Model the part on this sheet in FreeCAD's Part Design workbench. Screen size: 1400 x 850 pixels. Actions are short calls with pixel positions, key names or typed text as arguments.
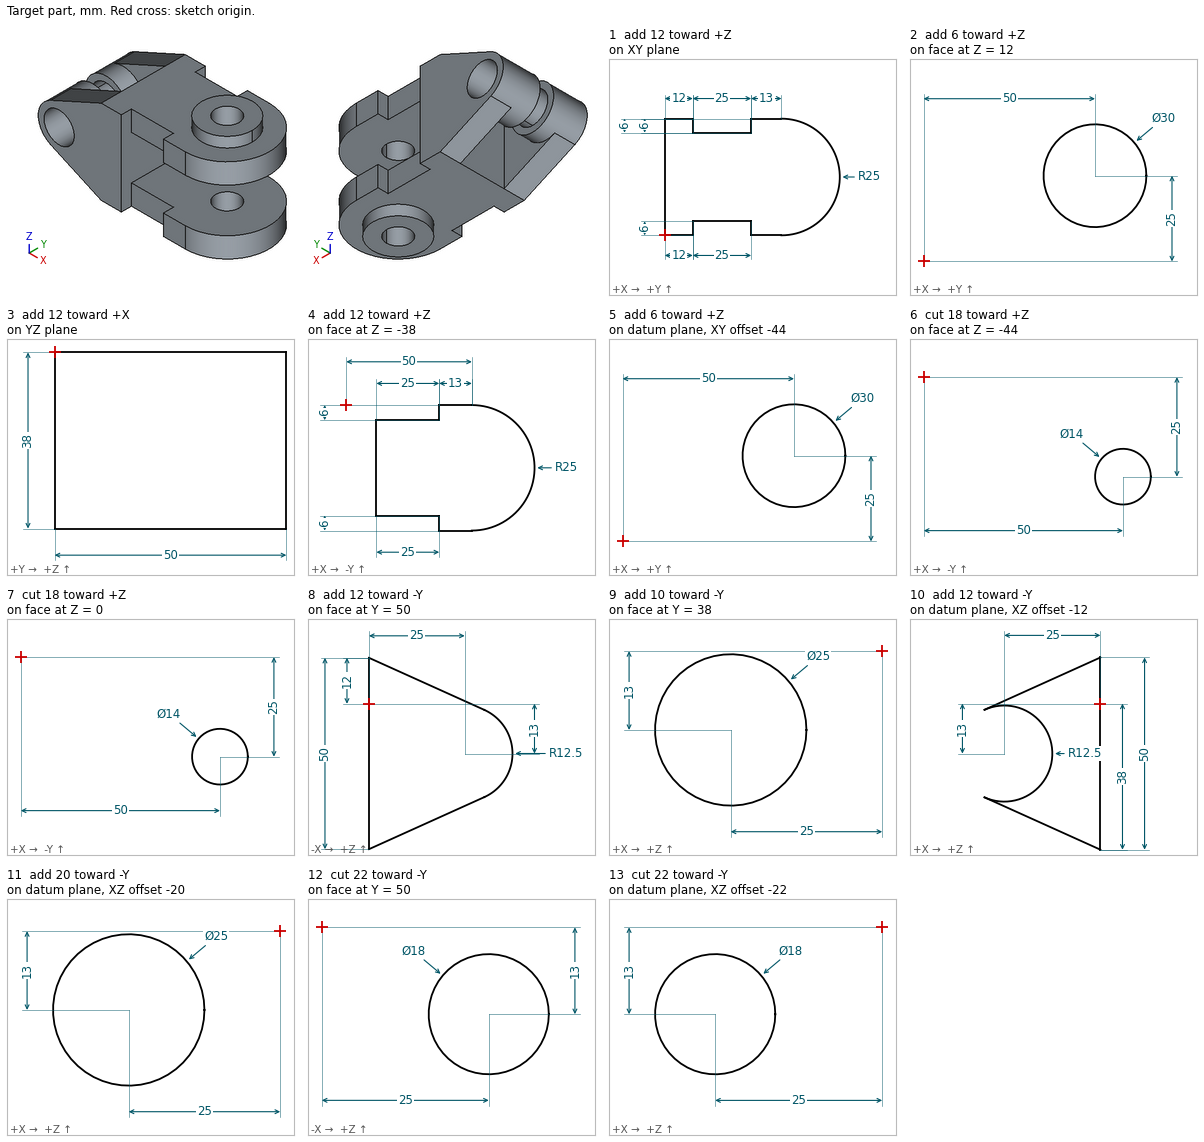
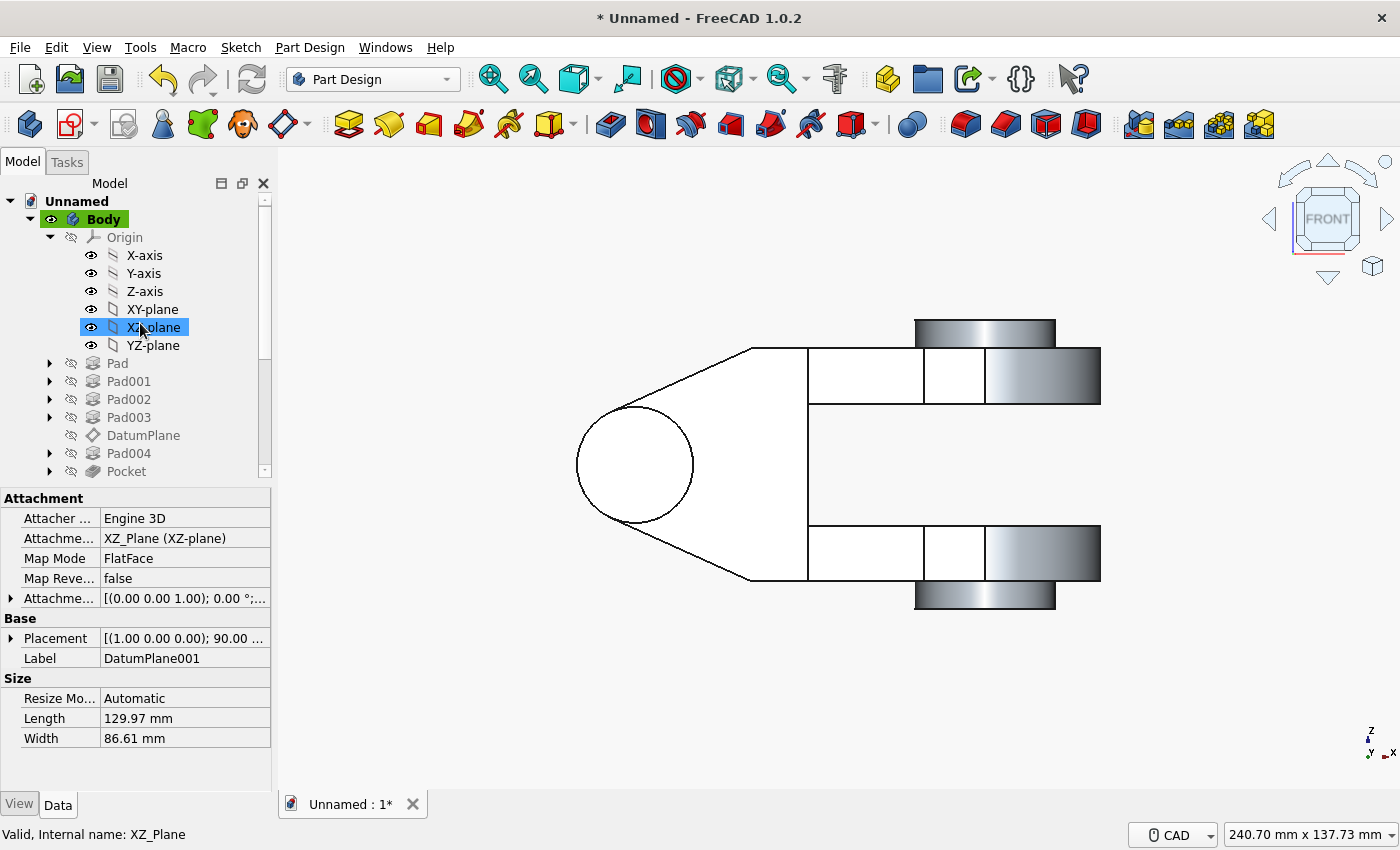
click(136, 327)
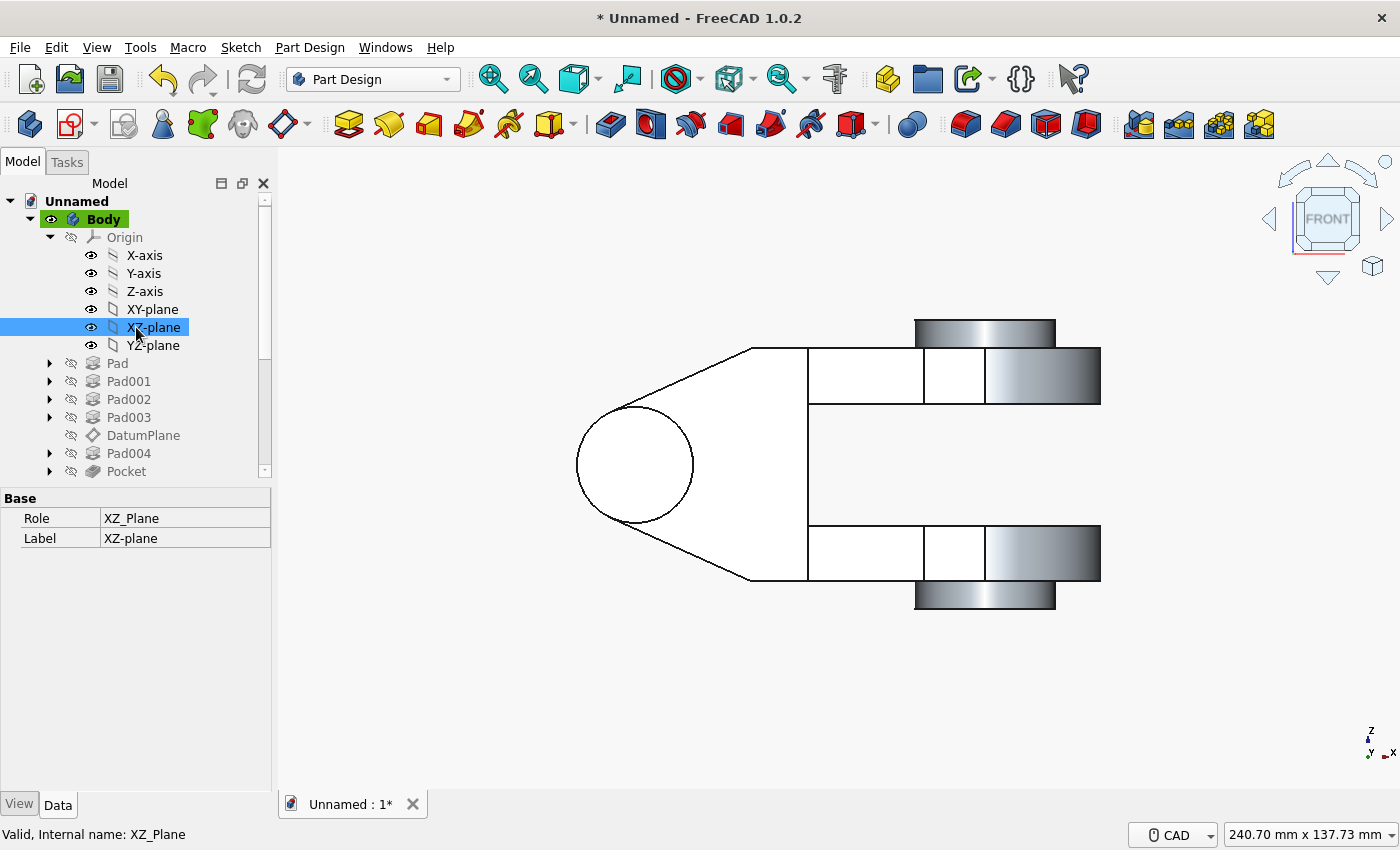
click(284, 124)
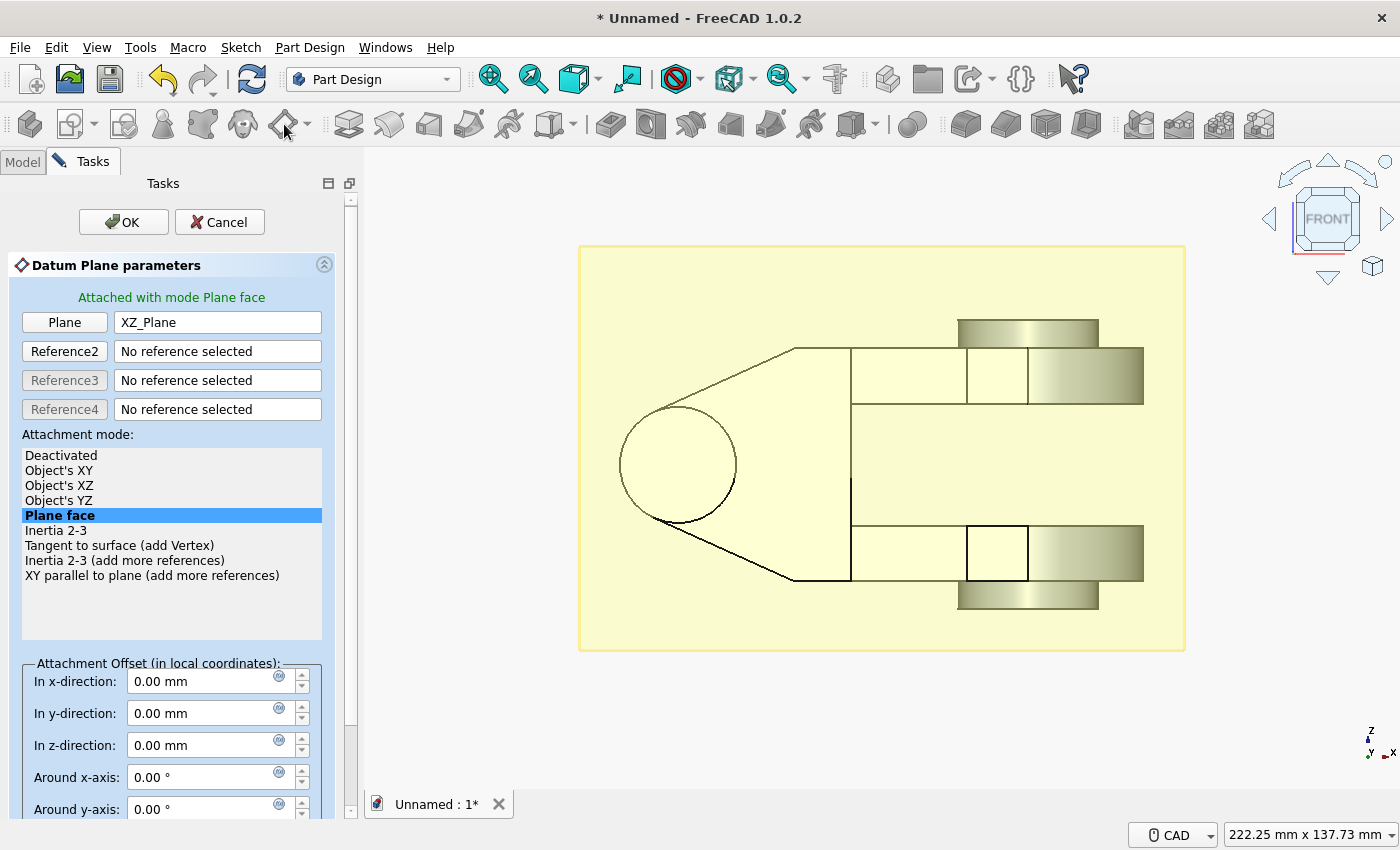
triple_click(210, 745)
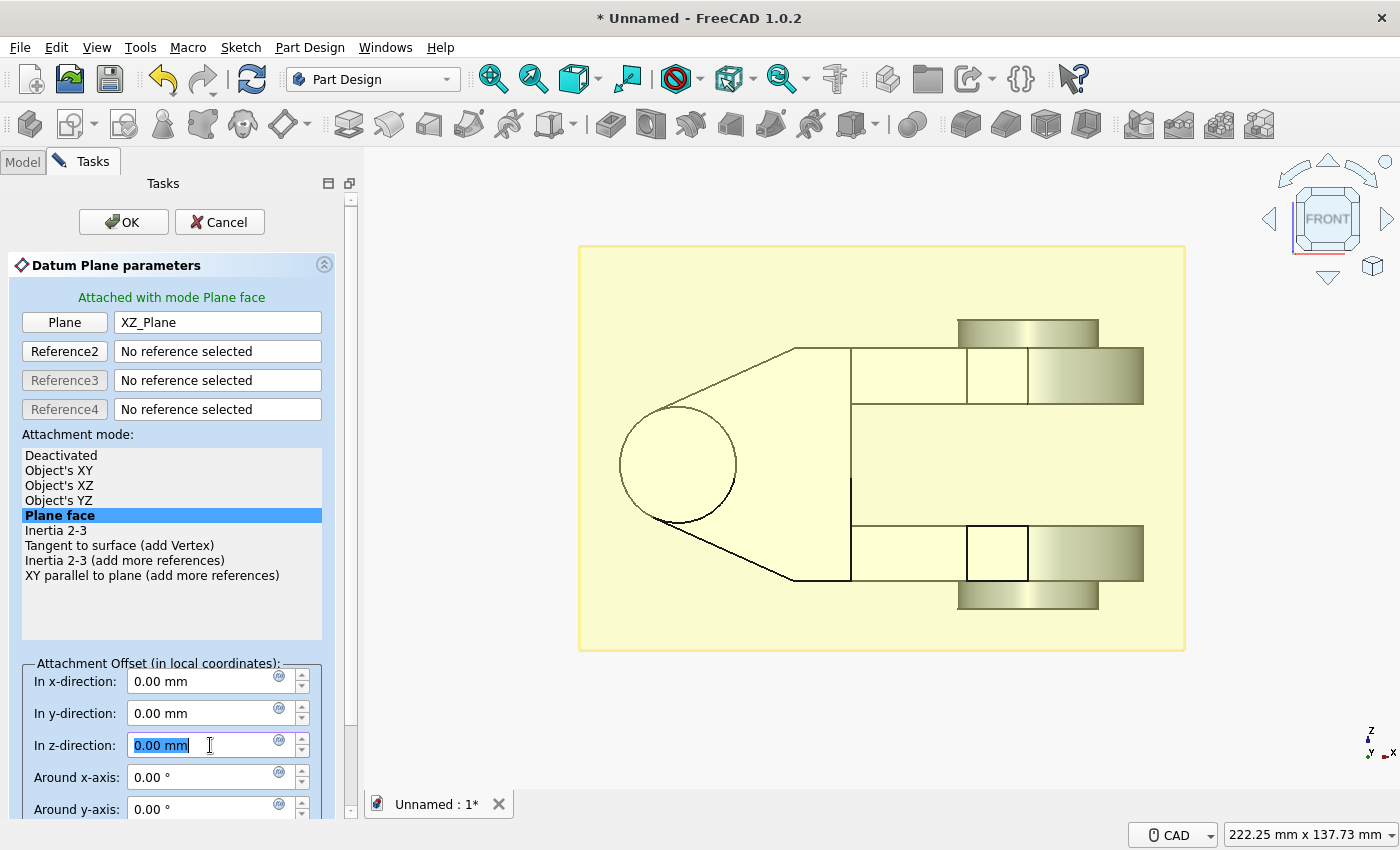
text(-20)
key(Tab)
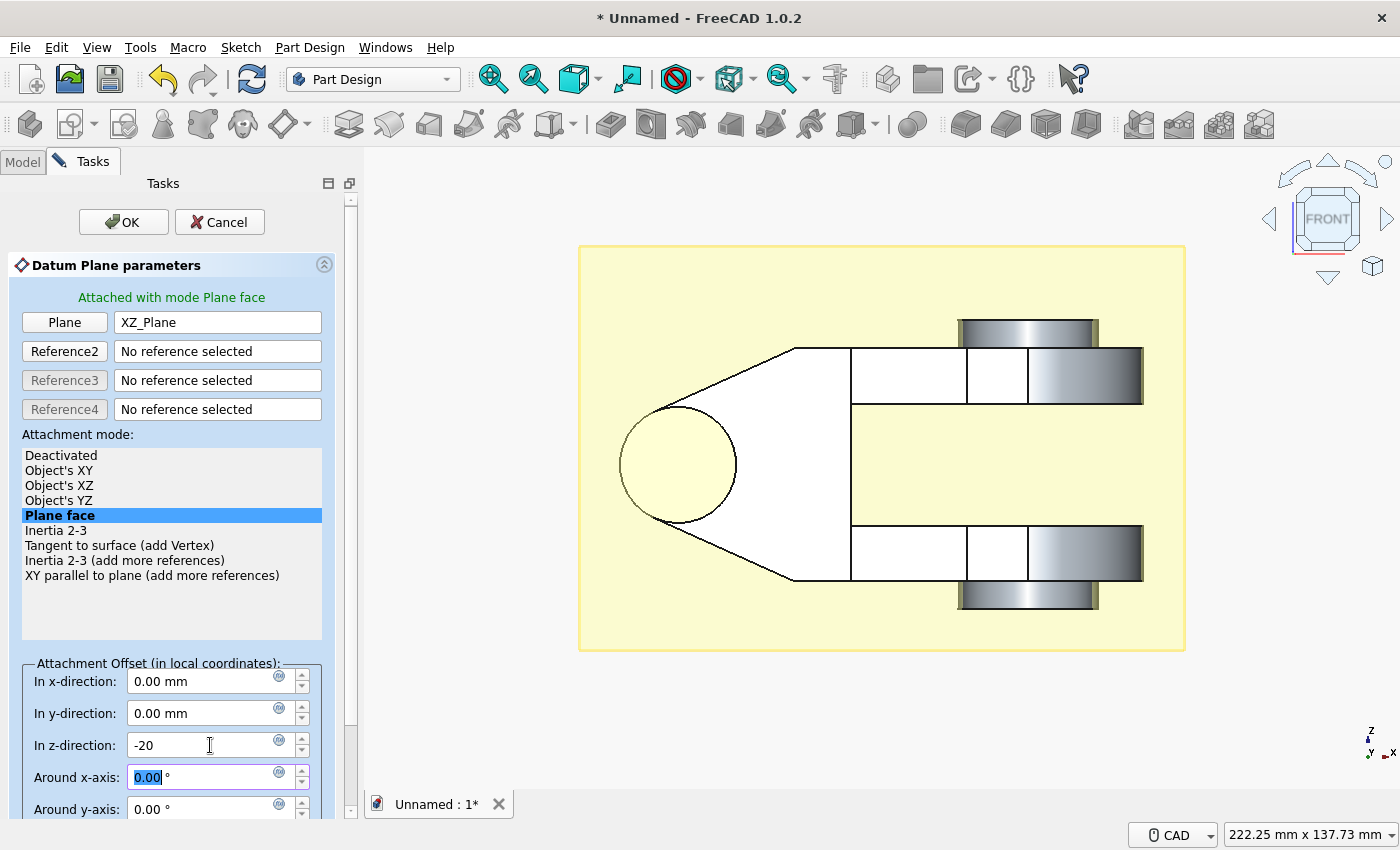
click(124, 222)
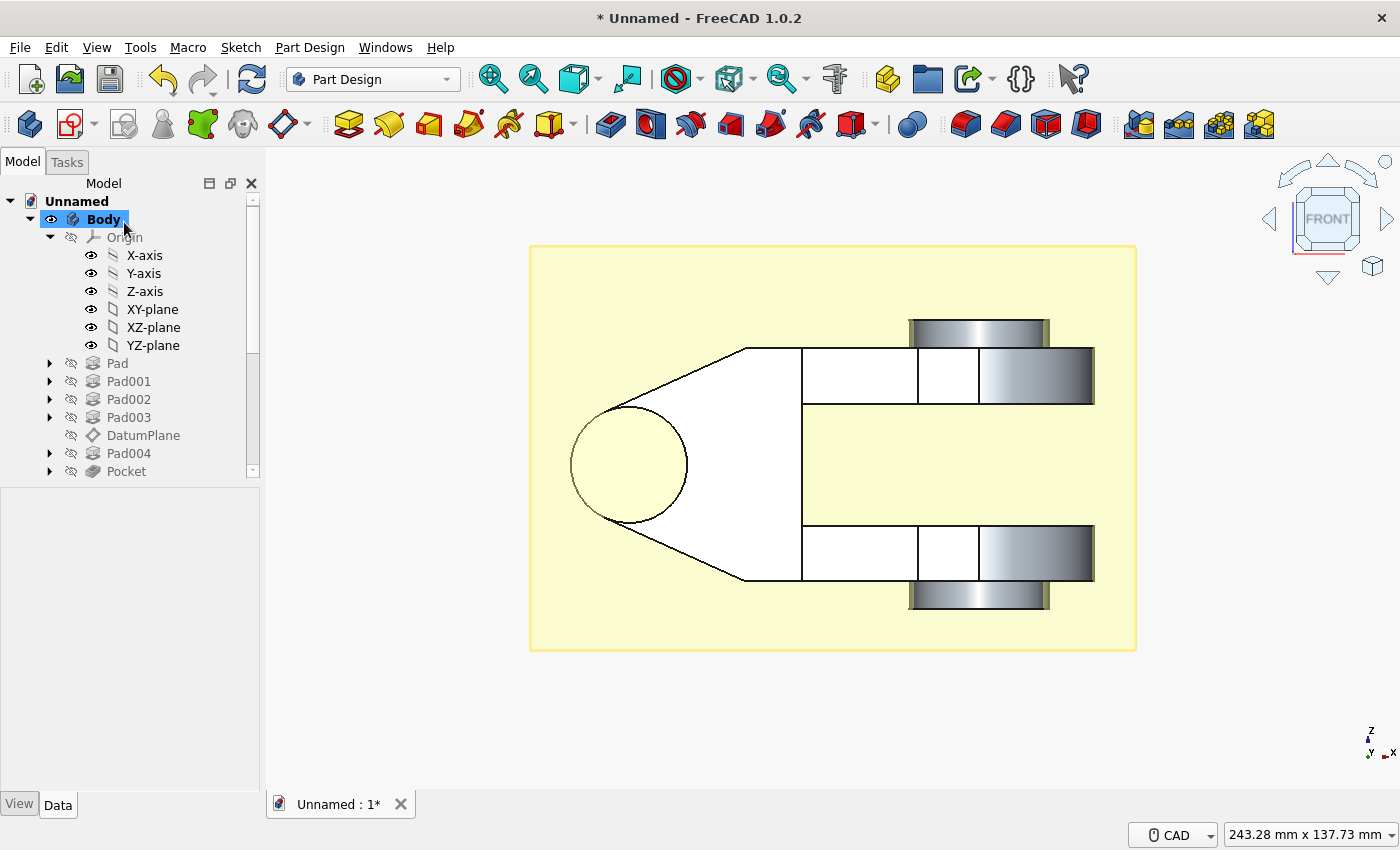
scroll(100, 341, down, 3)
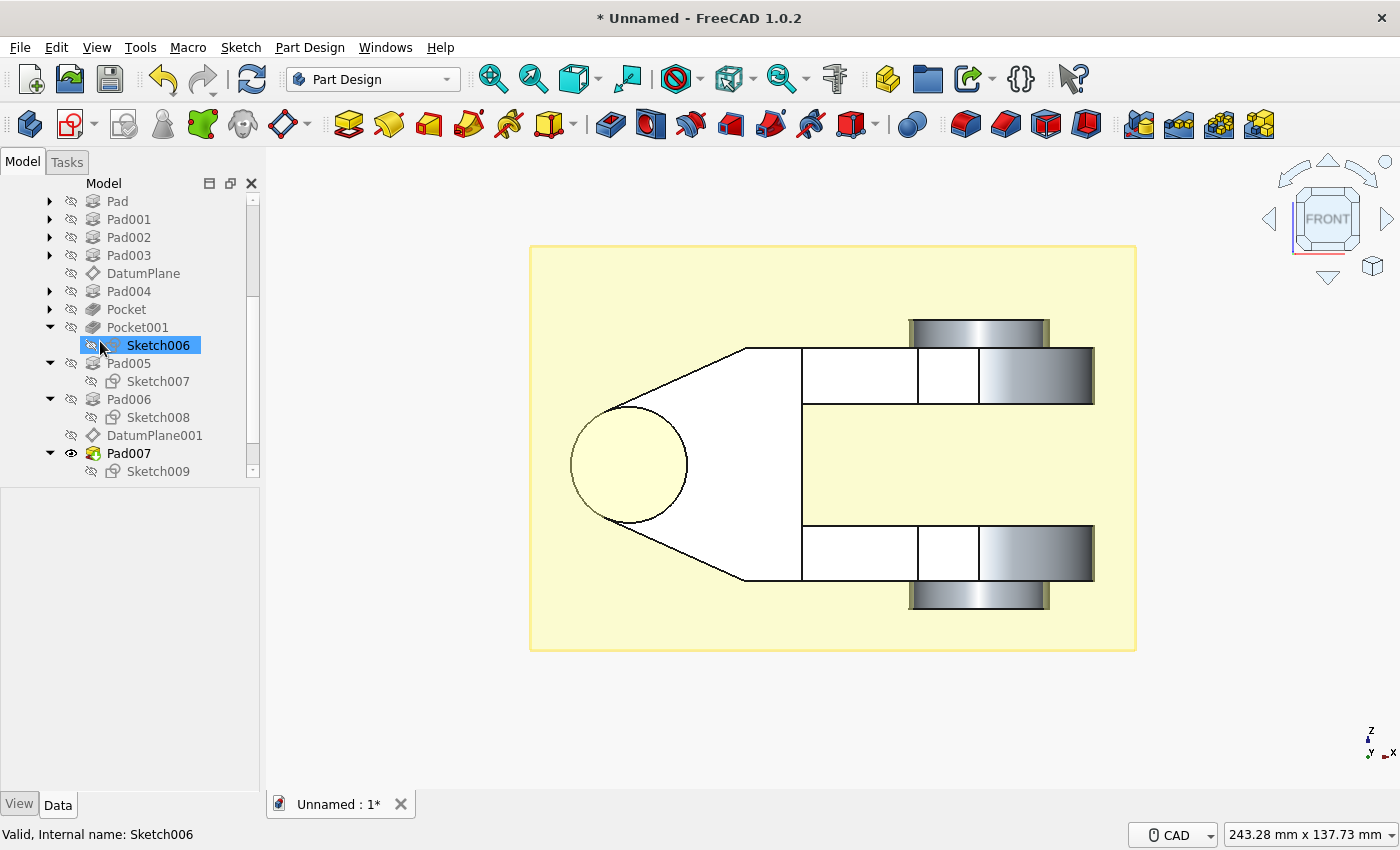
scroll(140, 341, up, 15)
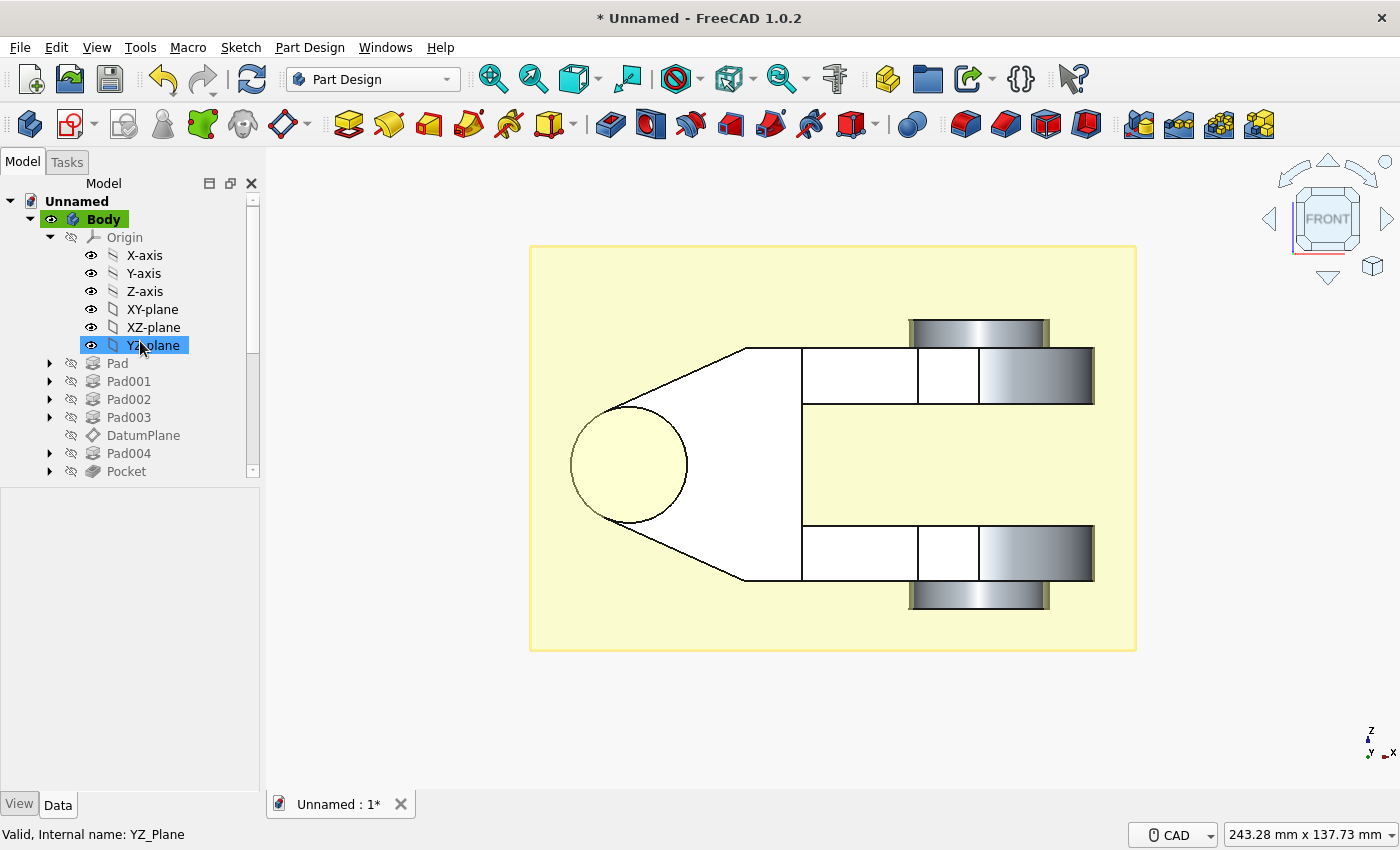
scroll(100, 341, down, 6)